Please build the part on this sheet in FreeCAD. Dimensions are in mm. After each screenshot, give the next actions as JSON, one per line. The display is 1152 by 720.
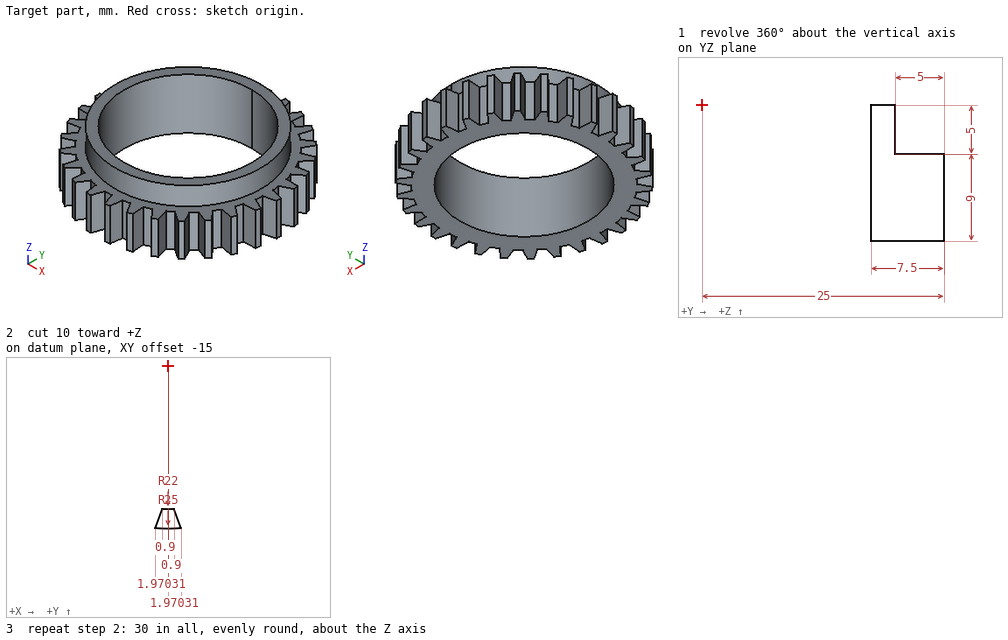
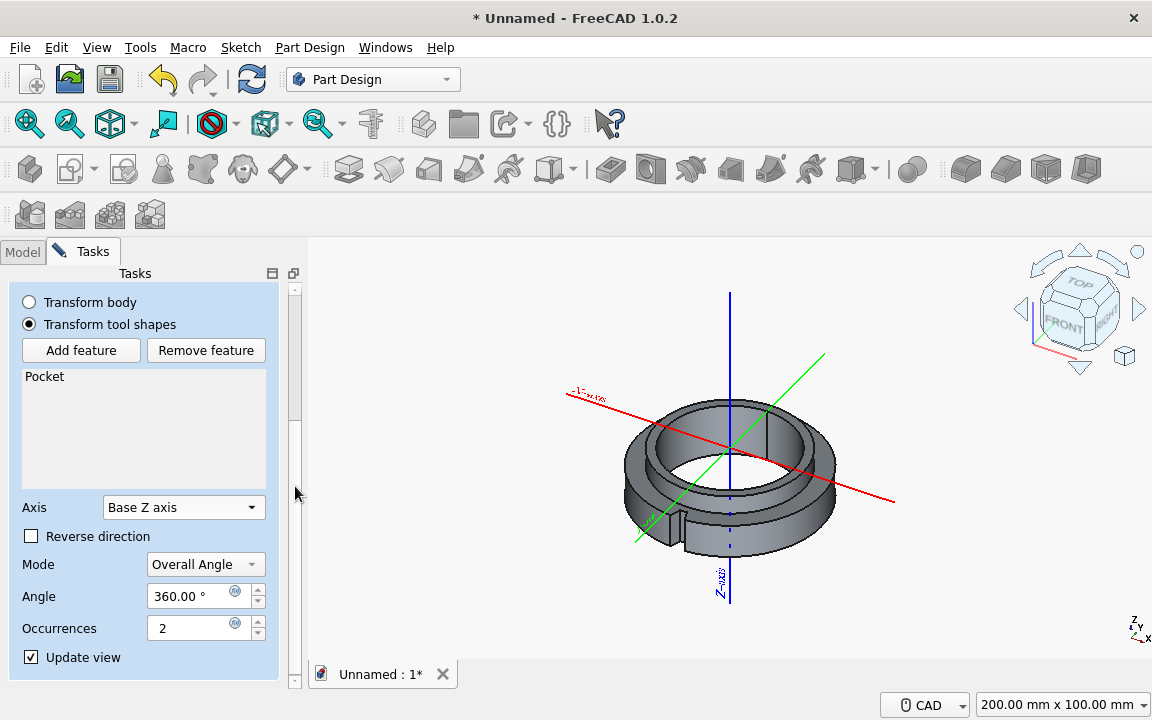
{"action": "triple_click", "coordinate": [198, 628]}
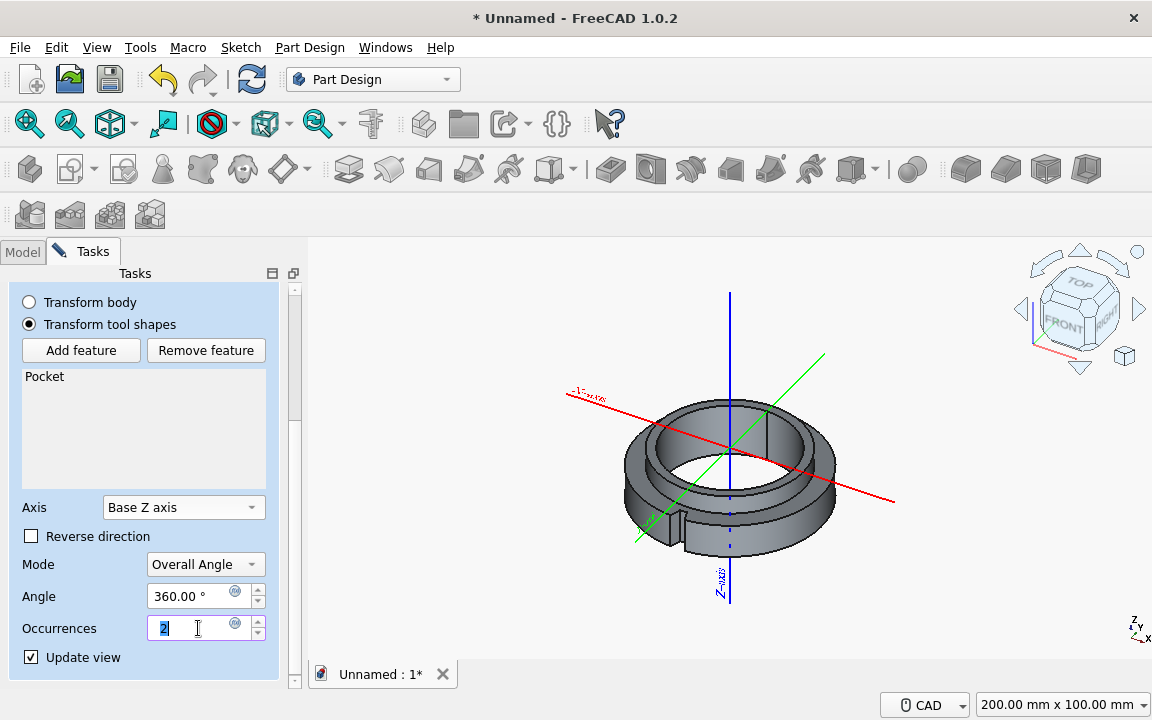
{"action": "type", "text": "30"}
{"action": "key", "text": "Tab"}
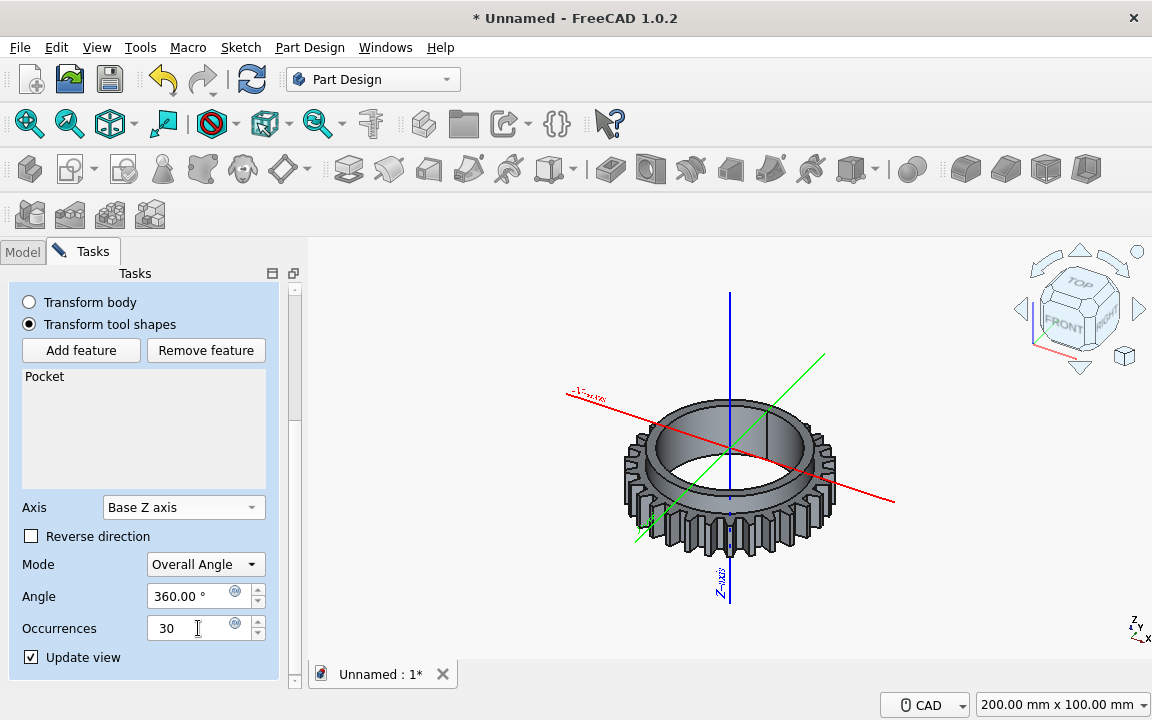
{"action": "scroll", "coordinate": [295, 486], "scroll_direction": "up", "scroll_amount": 5}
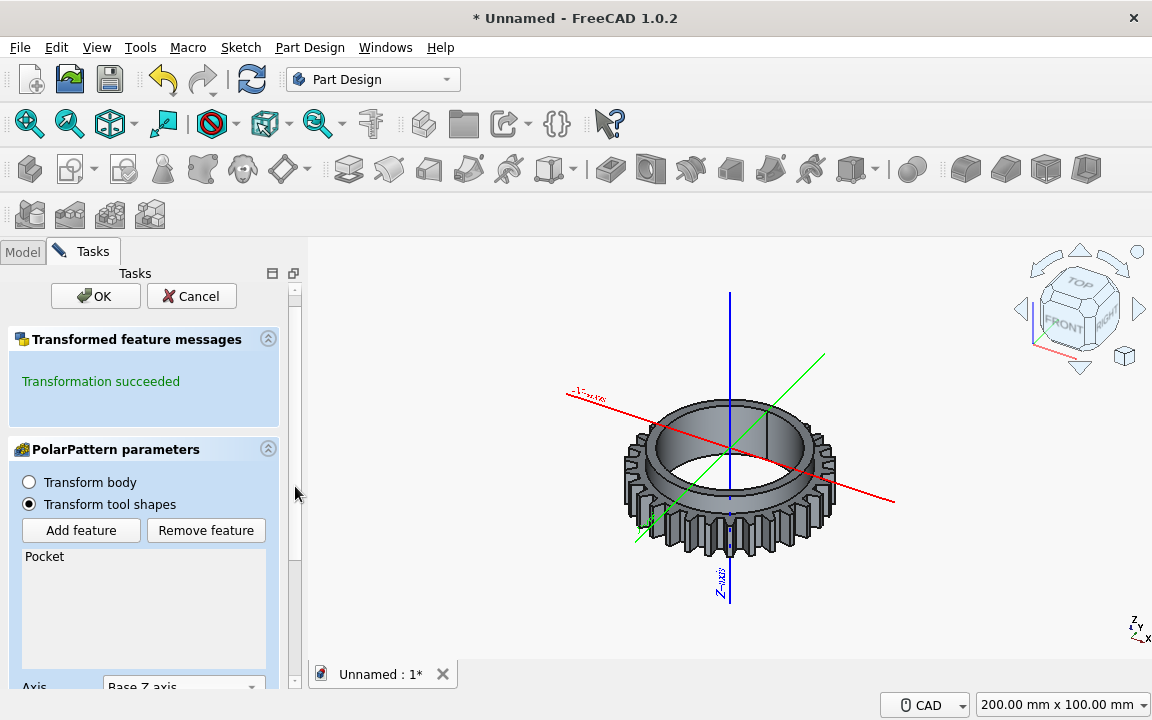
{"action": "left_click", "coordinate": [96, 312]}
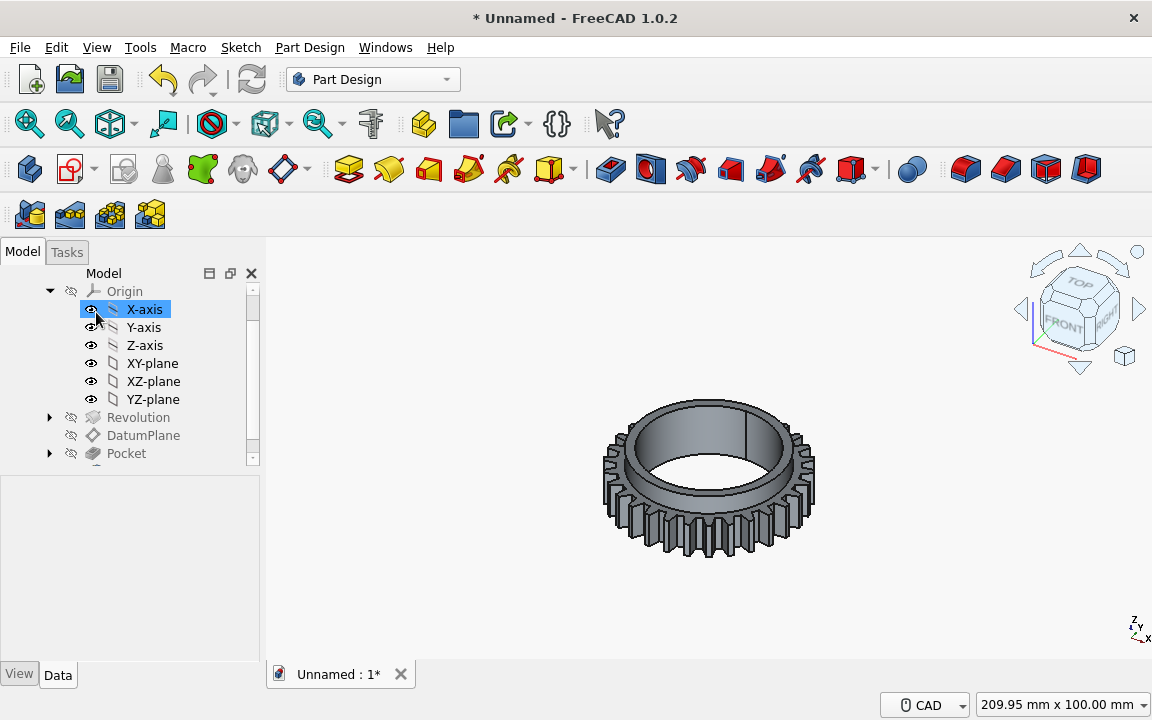
{"action": "key", "text": "0"}